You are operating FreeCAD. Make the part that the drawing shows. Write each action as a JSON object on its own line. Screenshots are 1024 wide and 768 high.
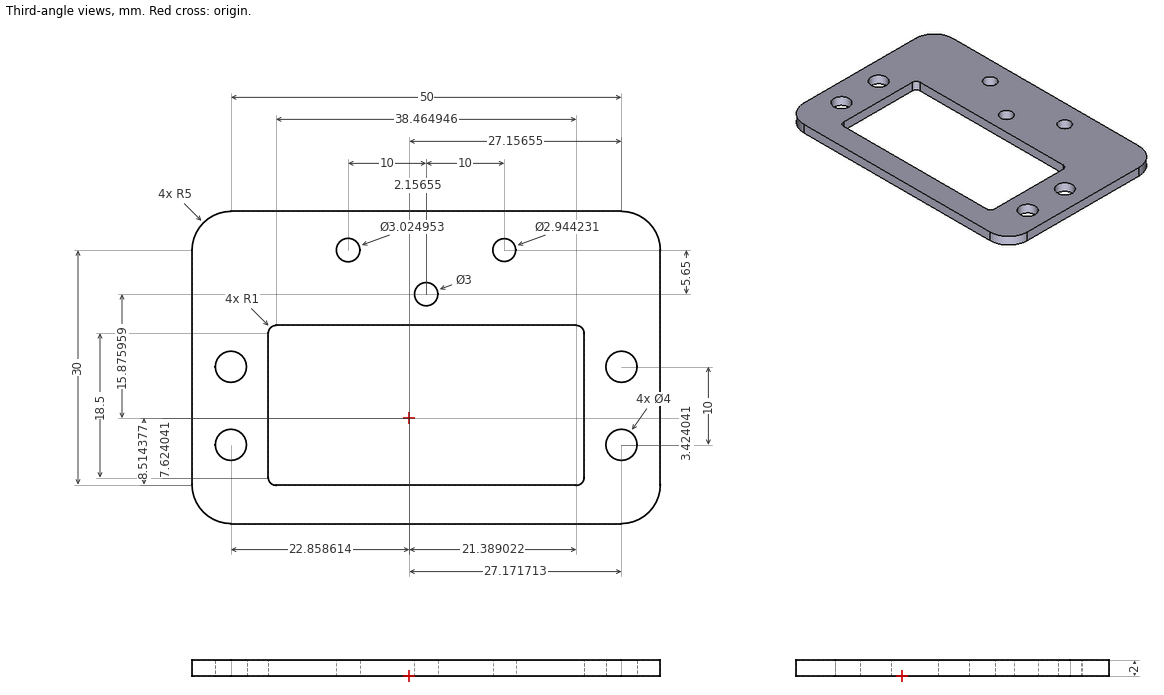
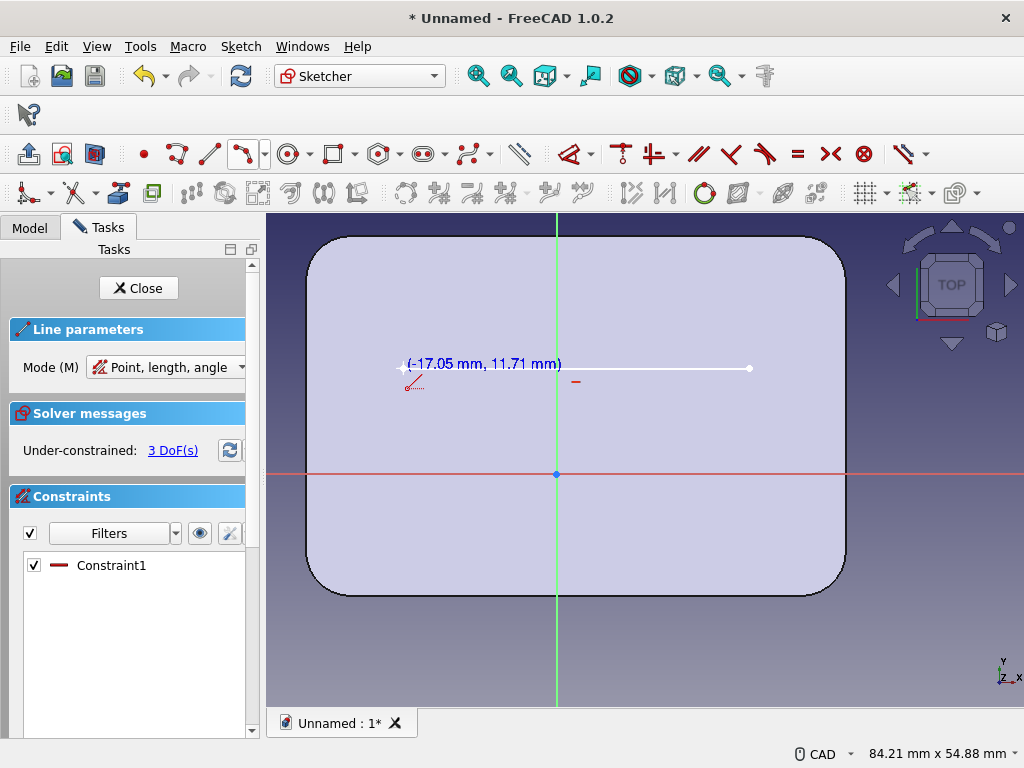
{"action": "scroll", "coordinate": [394, 377], "scroll_direction": "up", "scroll_amount": 2}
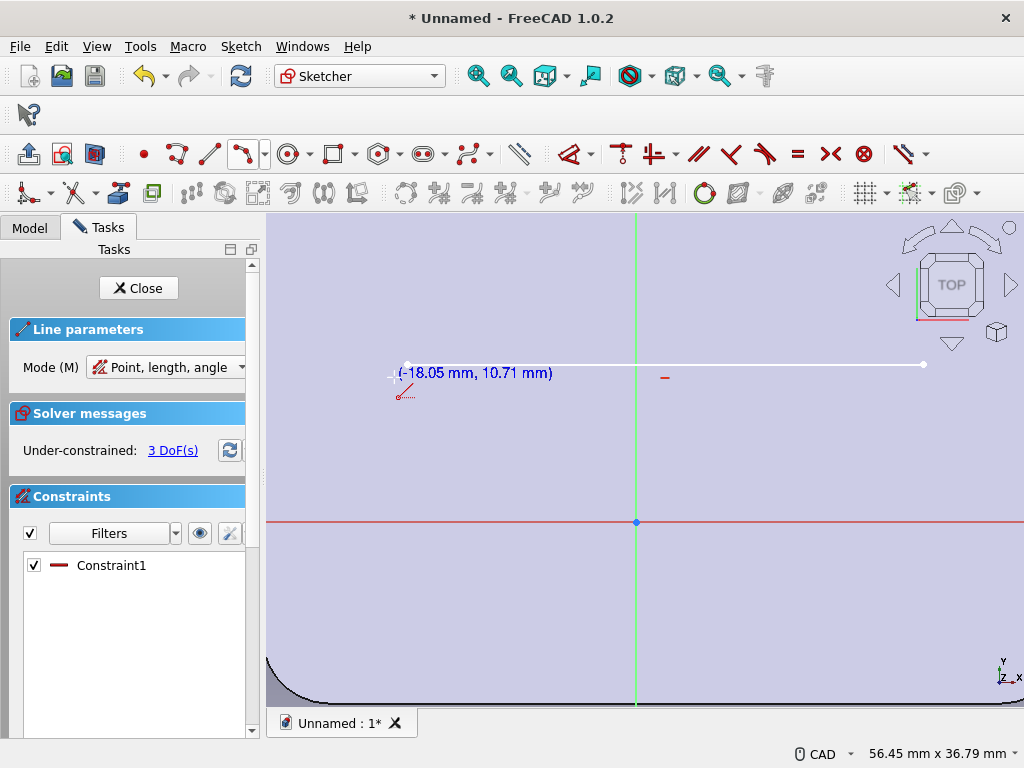
{"action": "left_click", "coordinate": [394, 376]}
{"action": "left_click", "coordinate": [394, 625]}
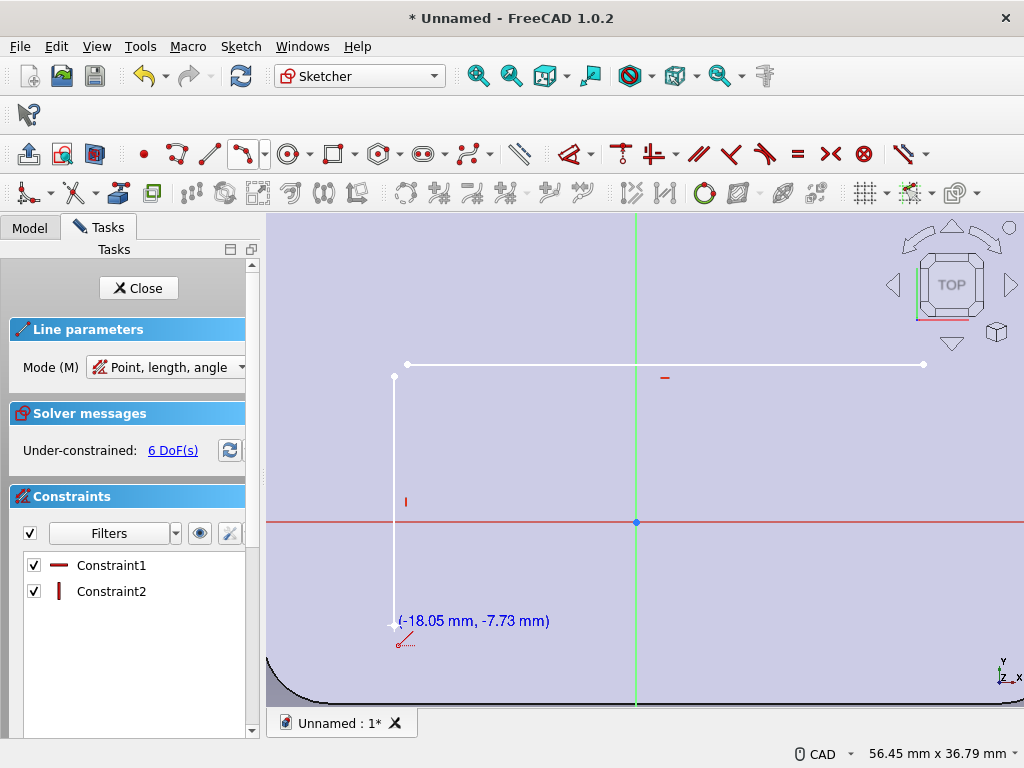
{"action": "left_click", "coordinate": [407, 638]}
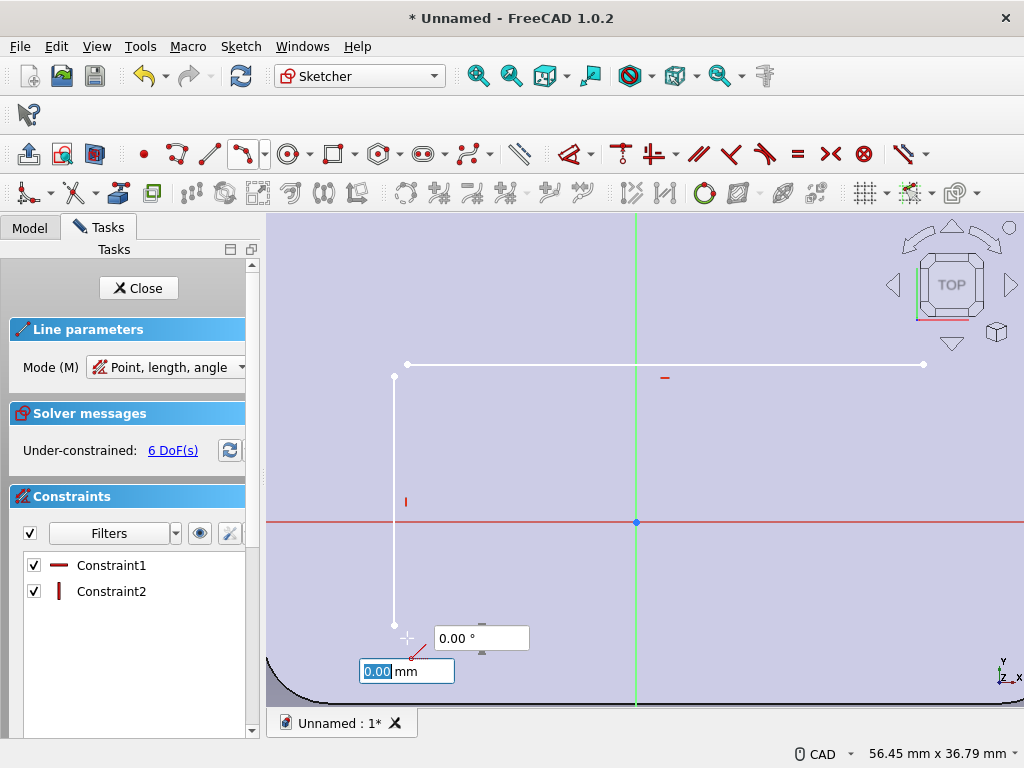
{"action": "scroll", "coordinate": [396, 378], "scroll_direction": "down", "scroll_amount": 2}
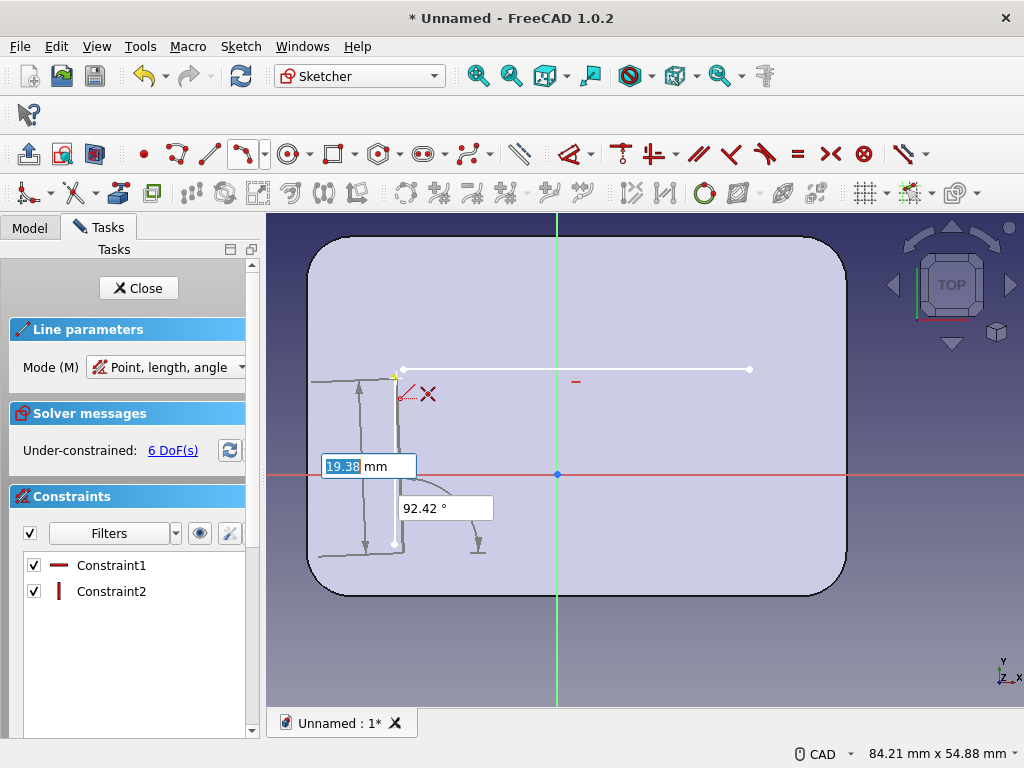
{"action": "left_click", "coordinate": [750, 552]}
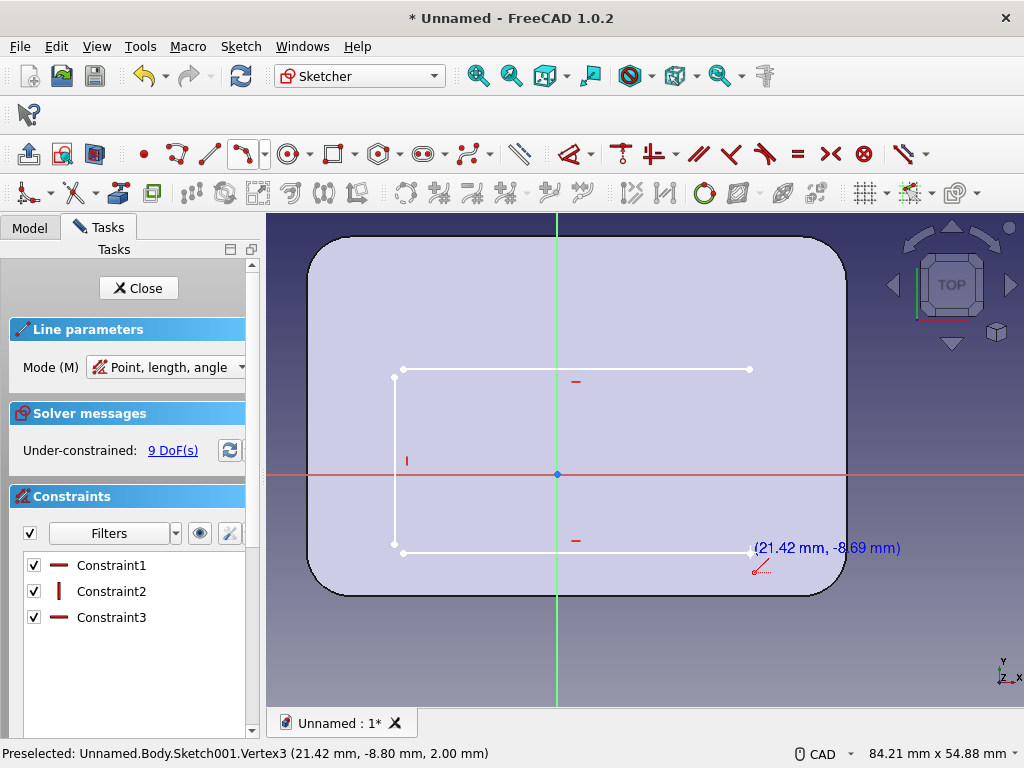
{"action": "scroll", "coordinate": [759, 543], "scroll_direction": "up", "scroll_amount": 2}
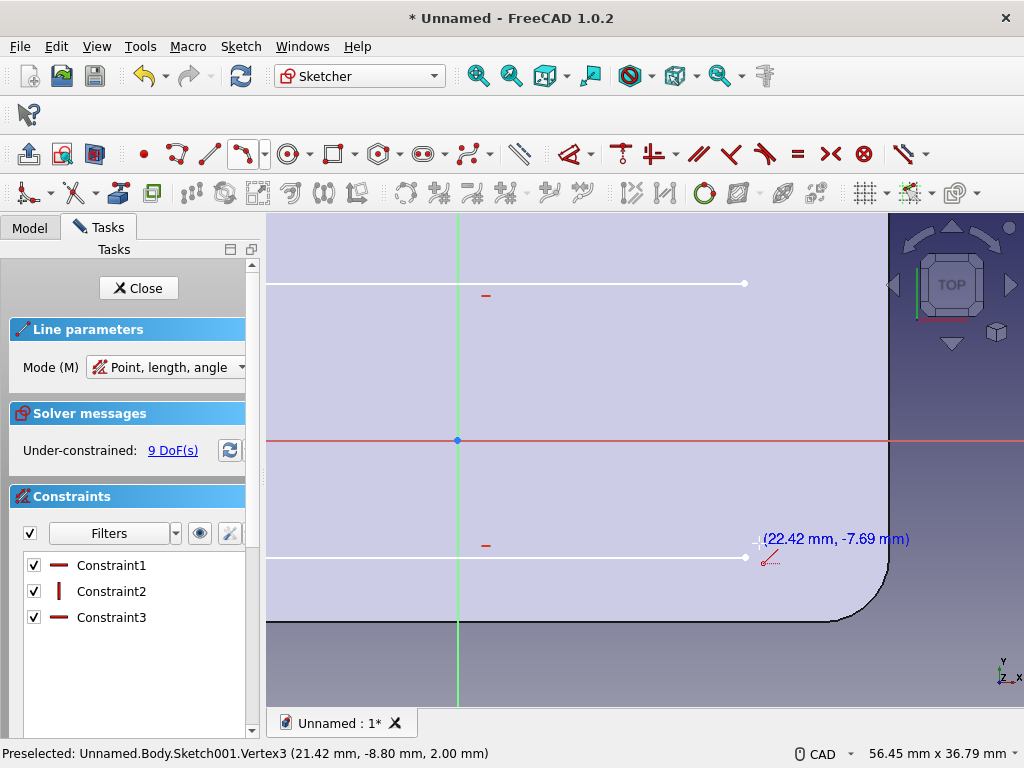
{"action": "left_click", "coordinate": [758, 543]}
{"action": "left_click", "coordinate": [758, 295]}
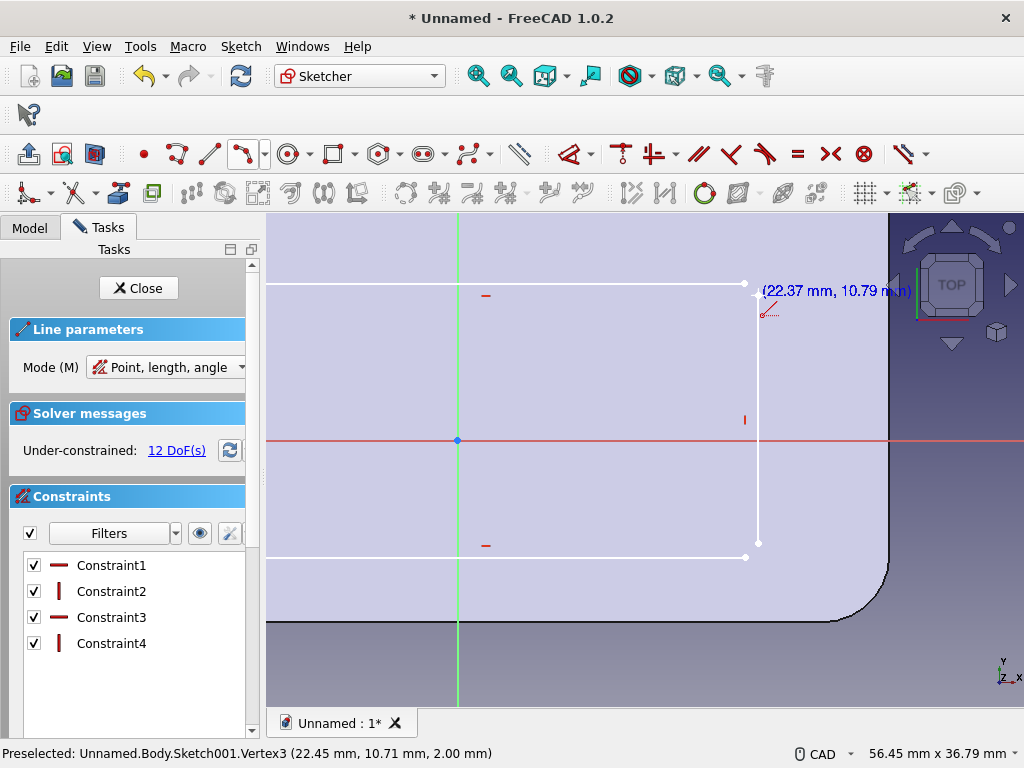
{"action": "left_click", "coordinate": [242, 154]}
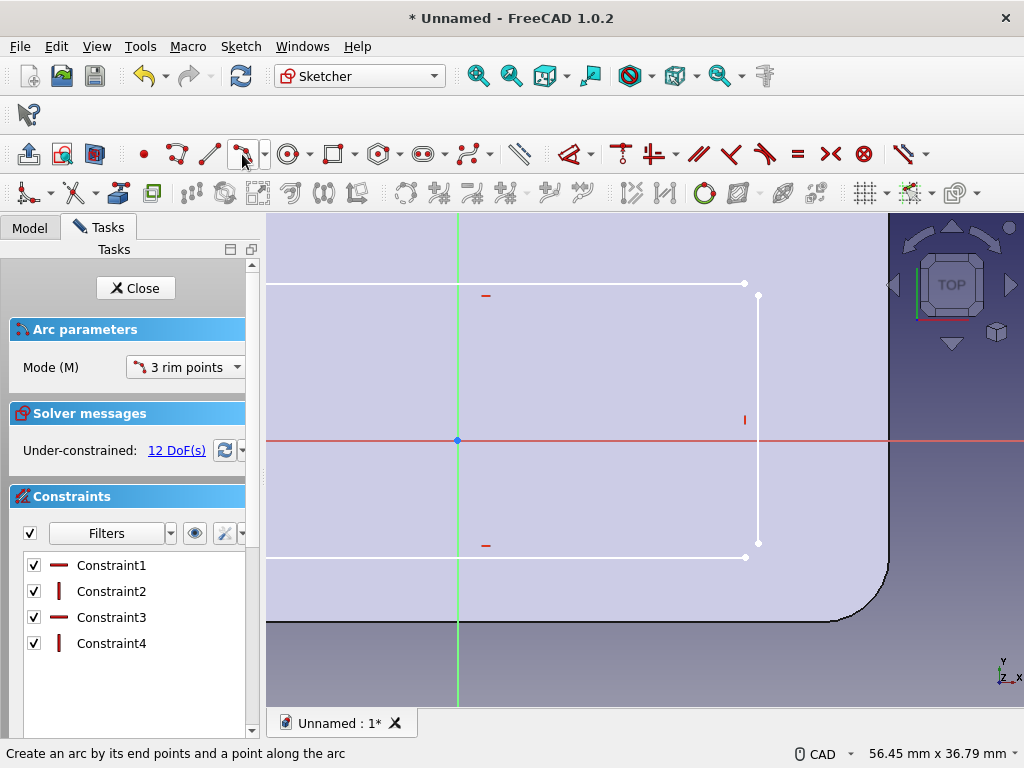
{"action": "scroll", "coordinate": [759, 543], "scroll_direction": "down", "scroll_amount": 2}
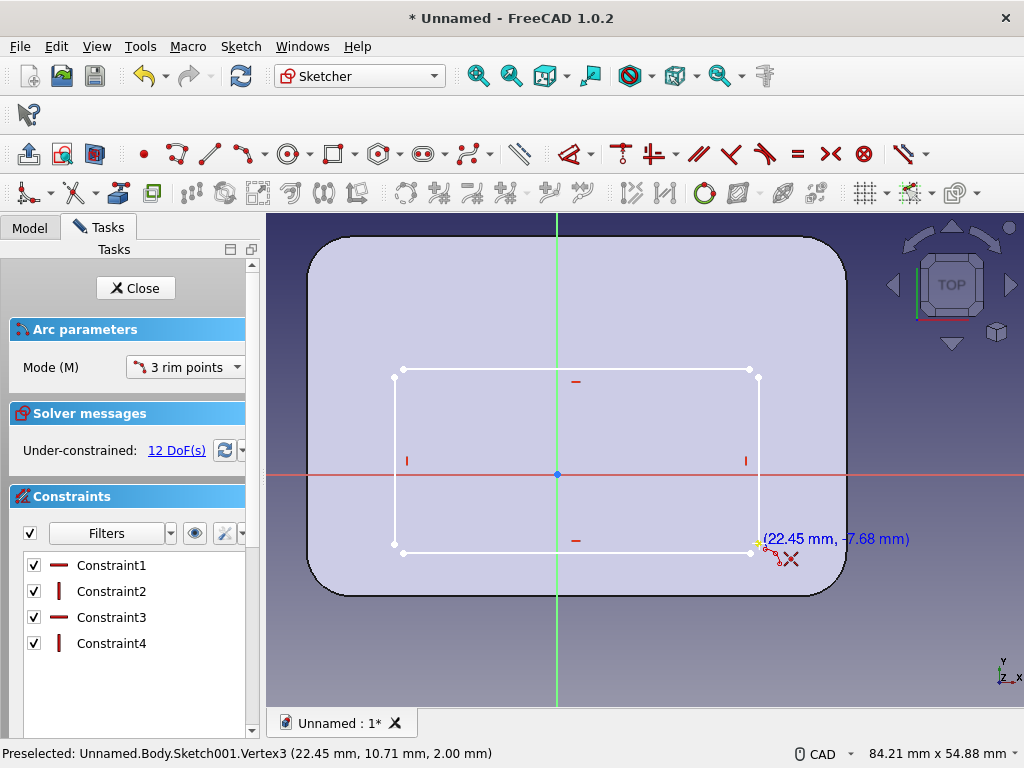
{"action": "scroll", "coordinate": [403, 368], "scroll_direction": "up", "scroll_amount": 2}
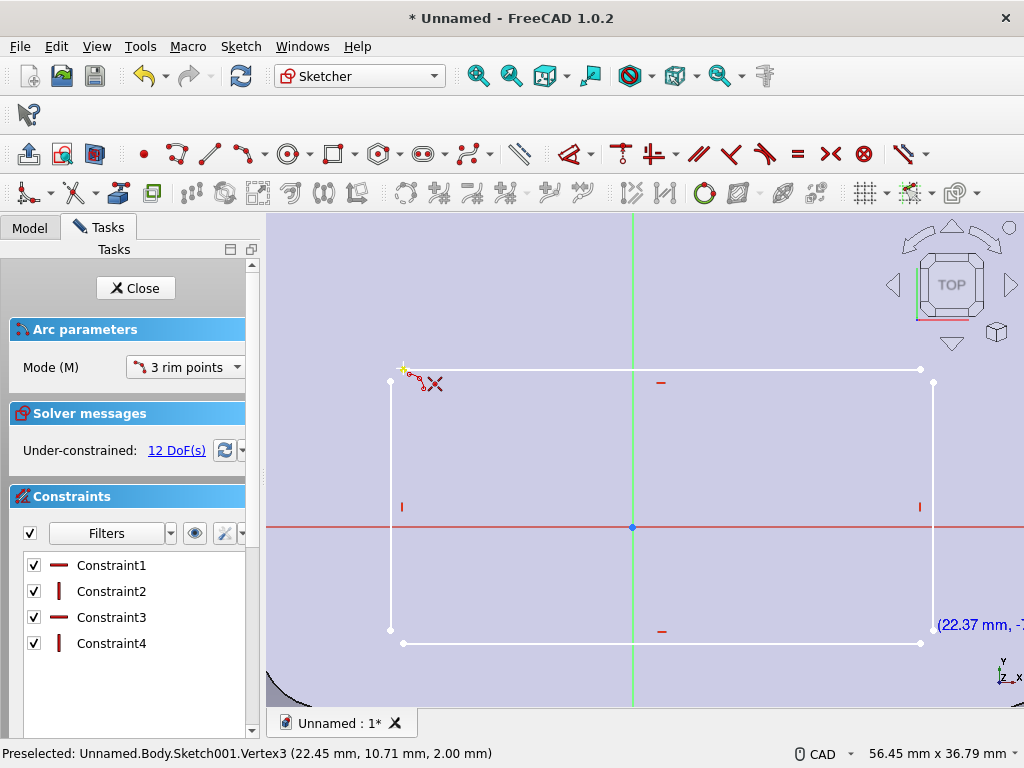
{"action": "left_click", "coordinate": [404, 370]}
{"action": "left_click", "coordinate": [391, 382]}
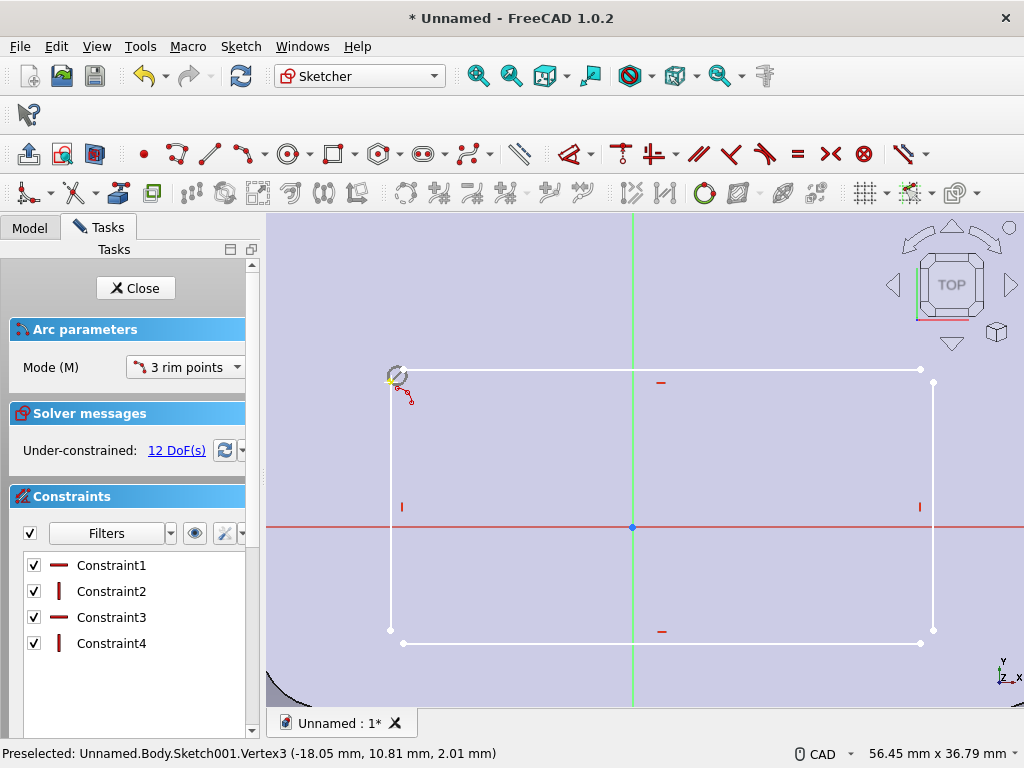
{"action": "scroll", "coordinate": [394, 372], "scroll_direction": "up", "scroll_amount": 7}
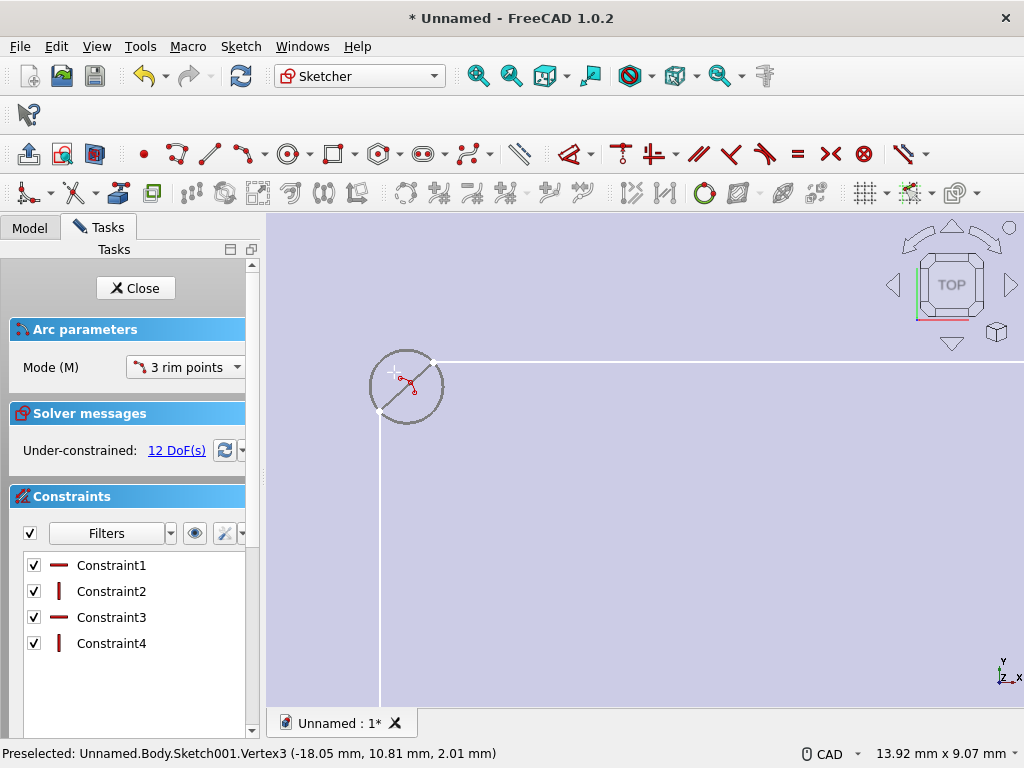
{"action": "left_click", "coordinate": [394, 369]}